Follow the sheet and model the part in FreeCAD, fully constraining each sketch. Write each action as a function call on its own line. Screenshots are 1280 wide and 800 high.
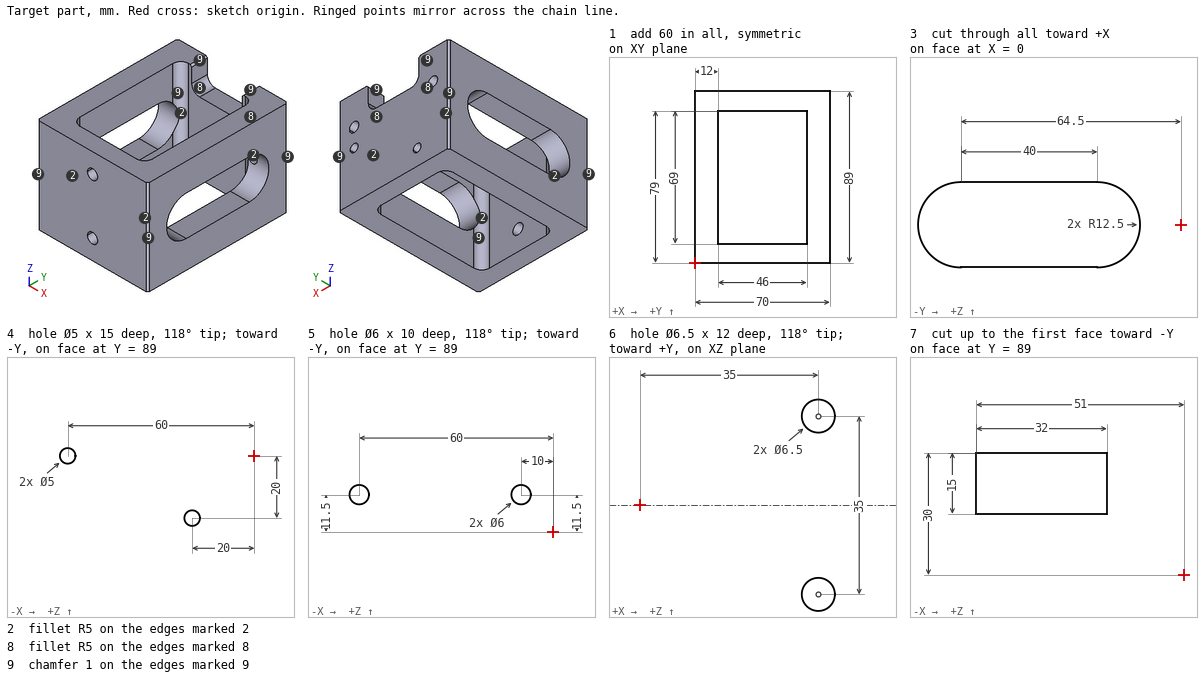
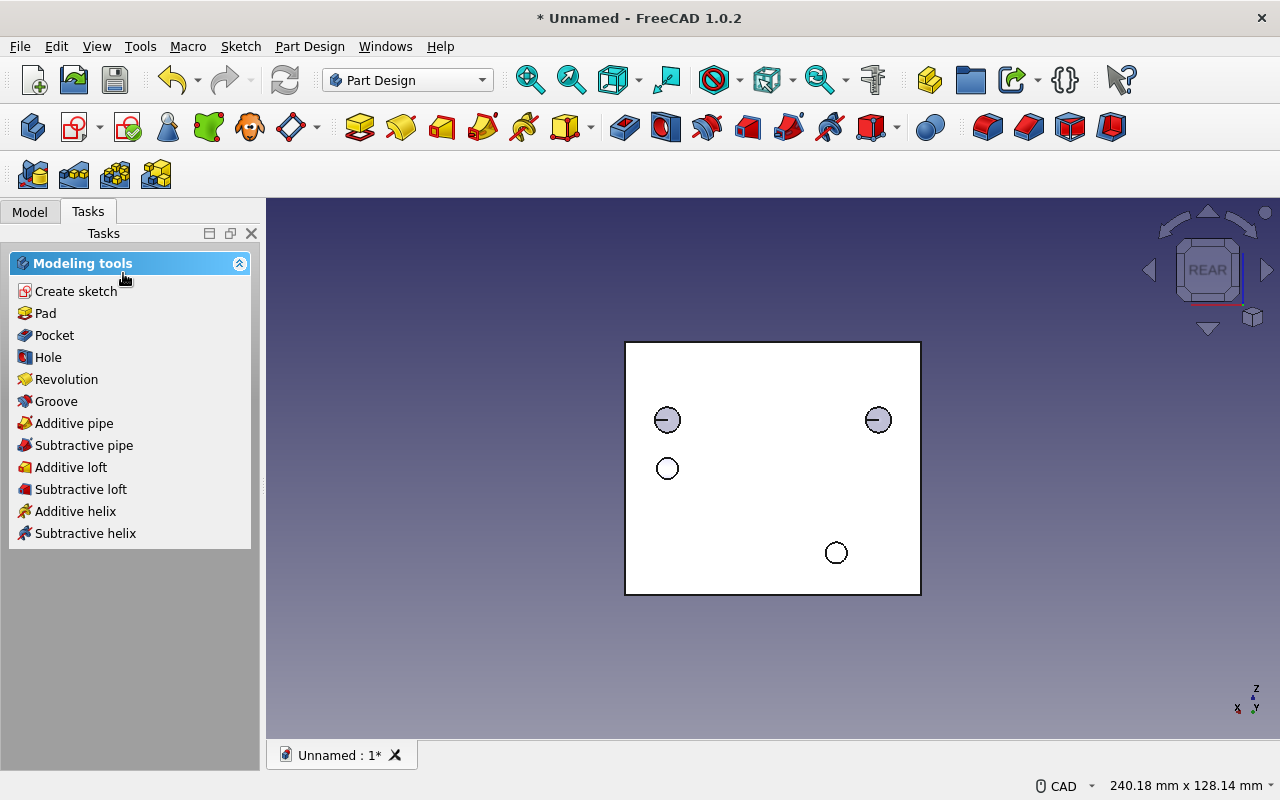
click(666, 128)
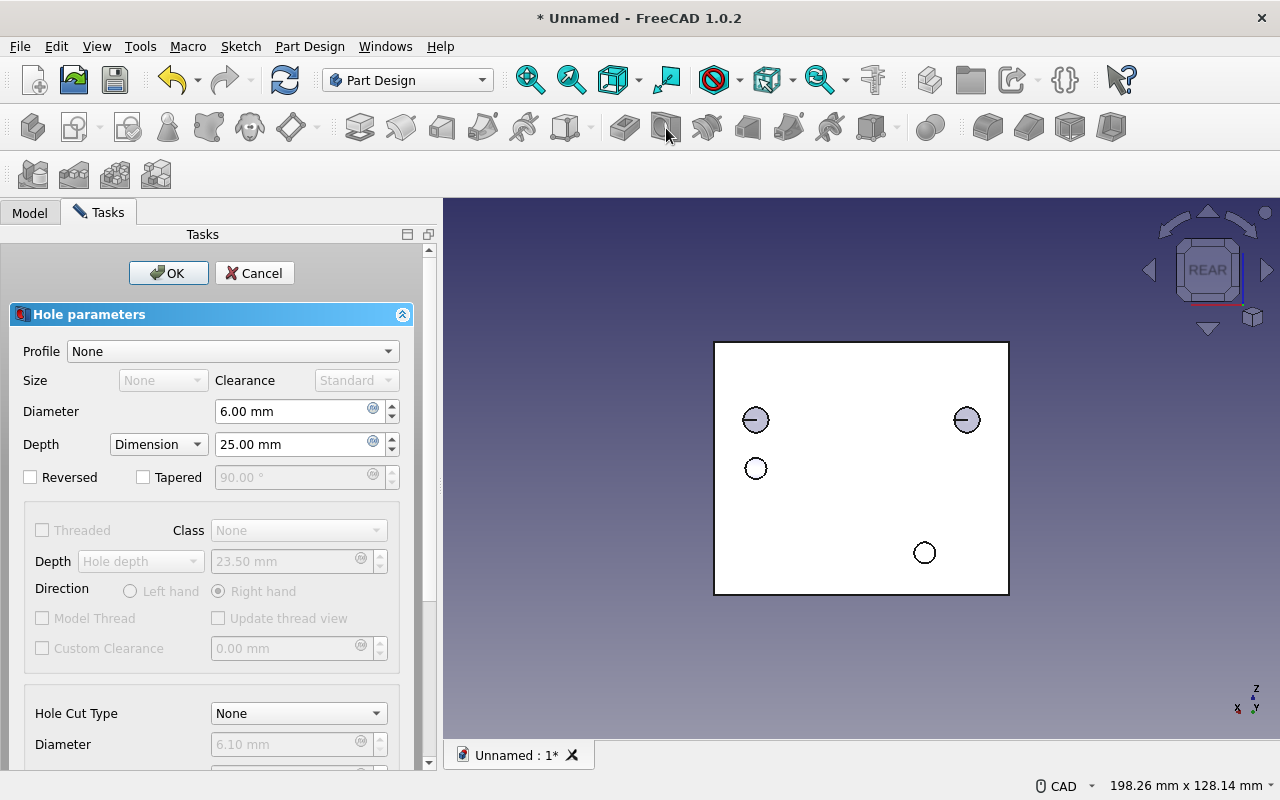
triple_click(300, 412)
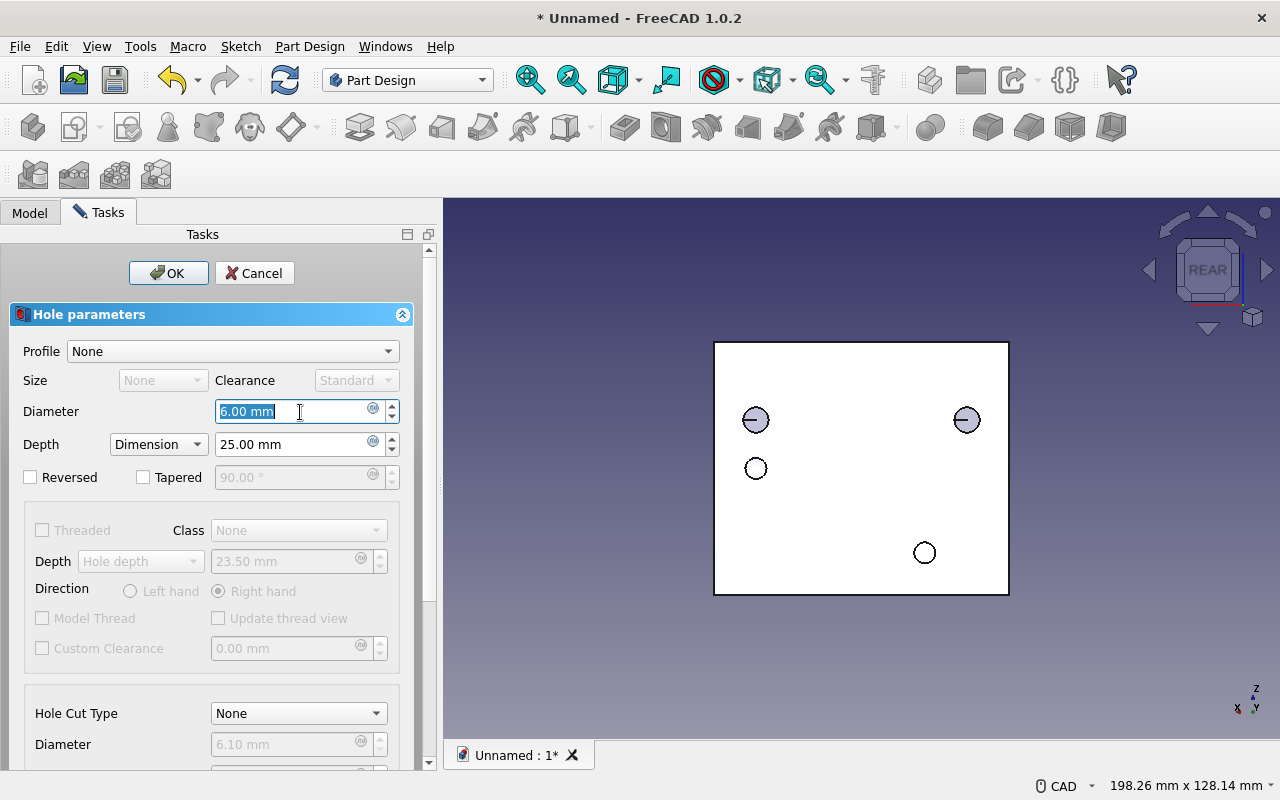
text(6.5)
key(Tab)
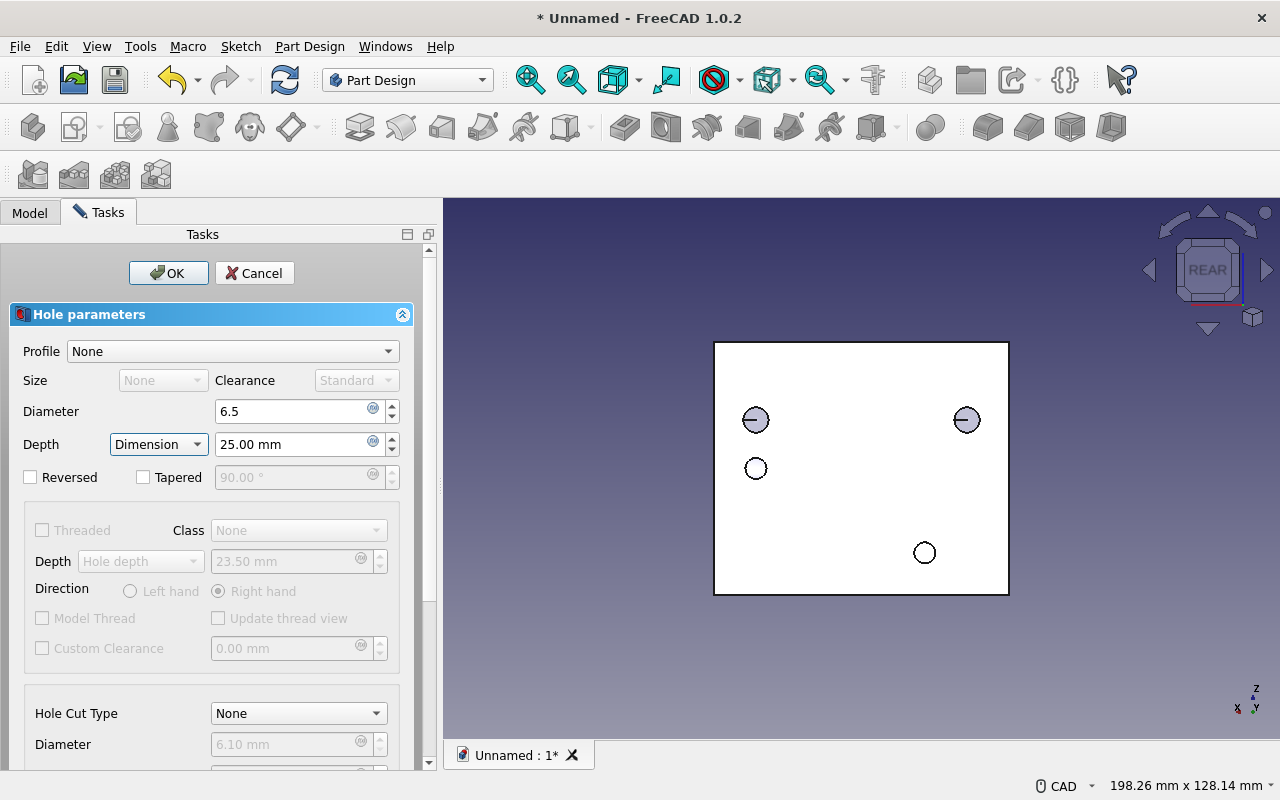
triple_click(300, 444)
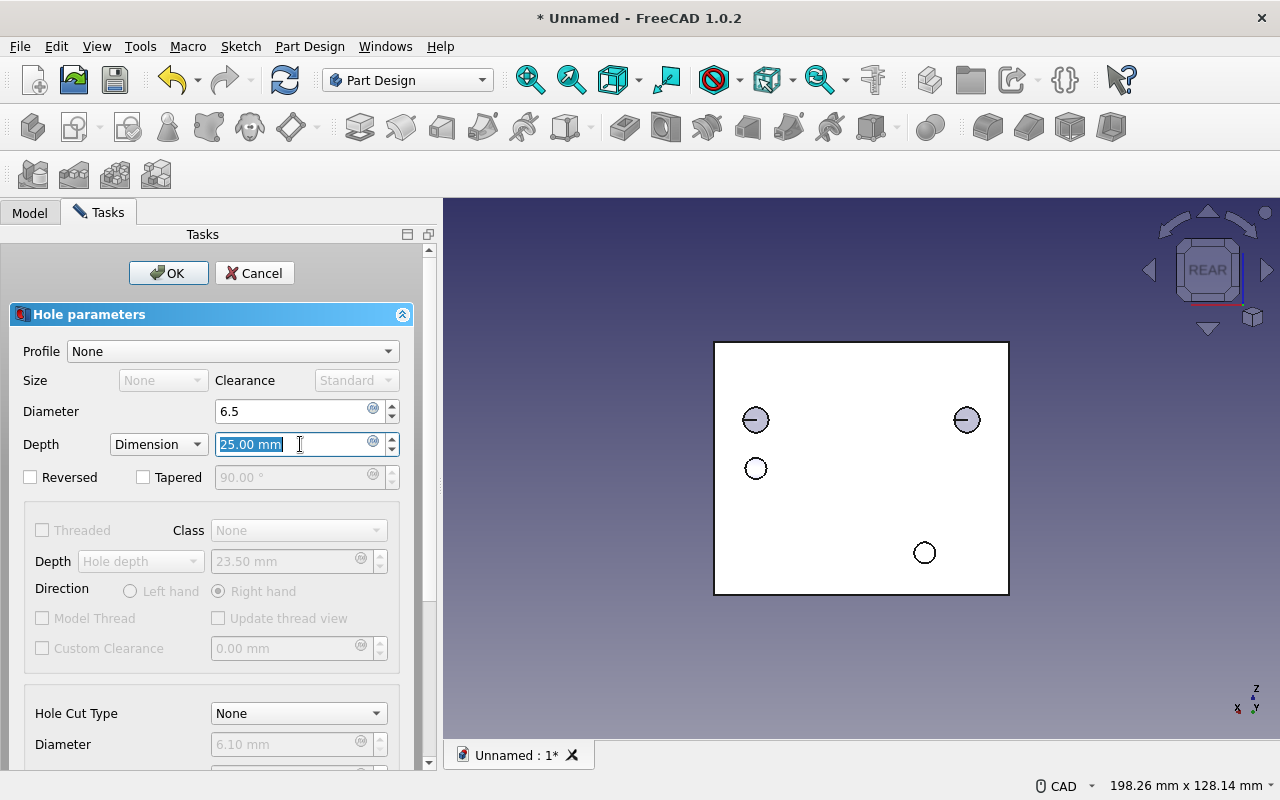
text(12)
key(Tab)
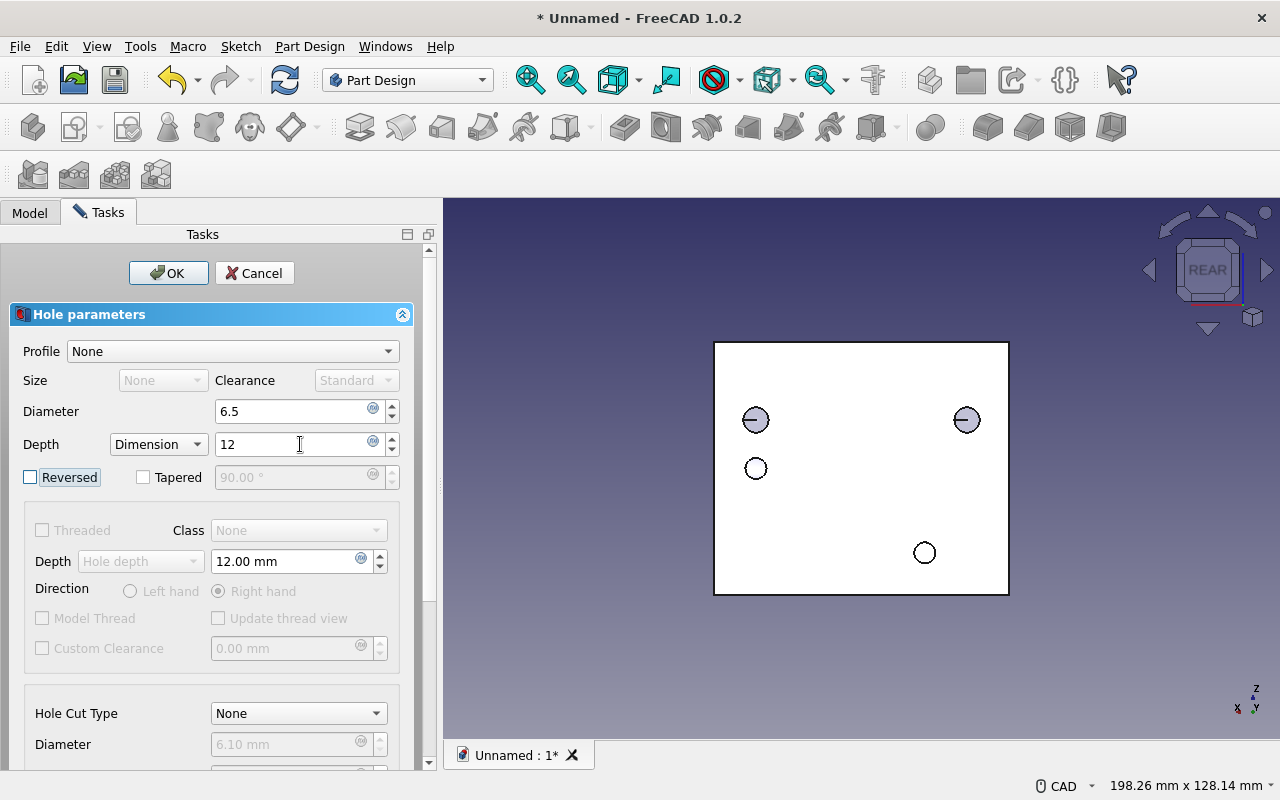
click(169, 273)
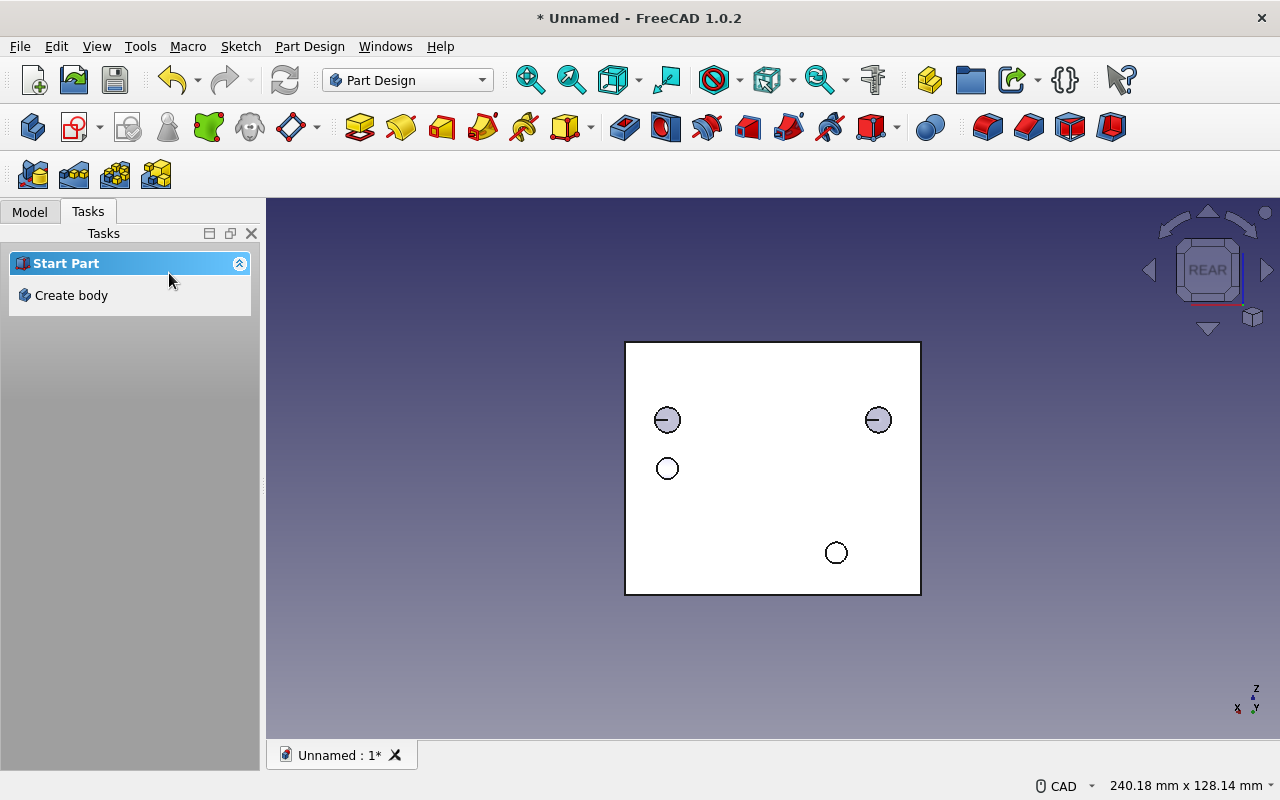
click(773, 468)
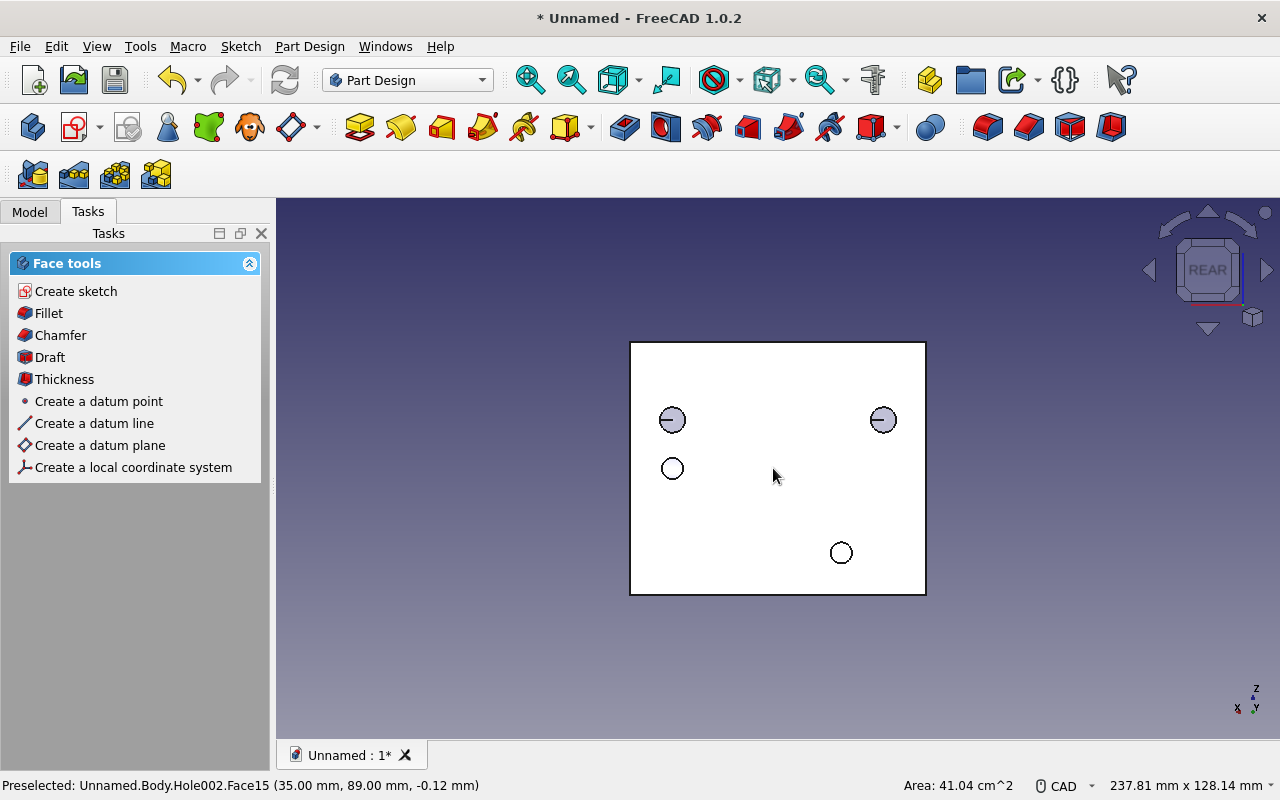
click(74, 128)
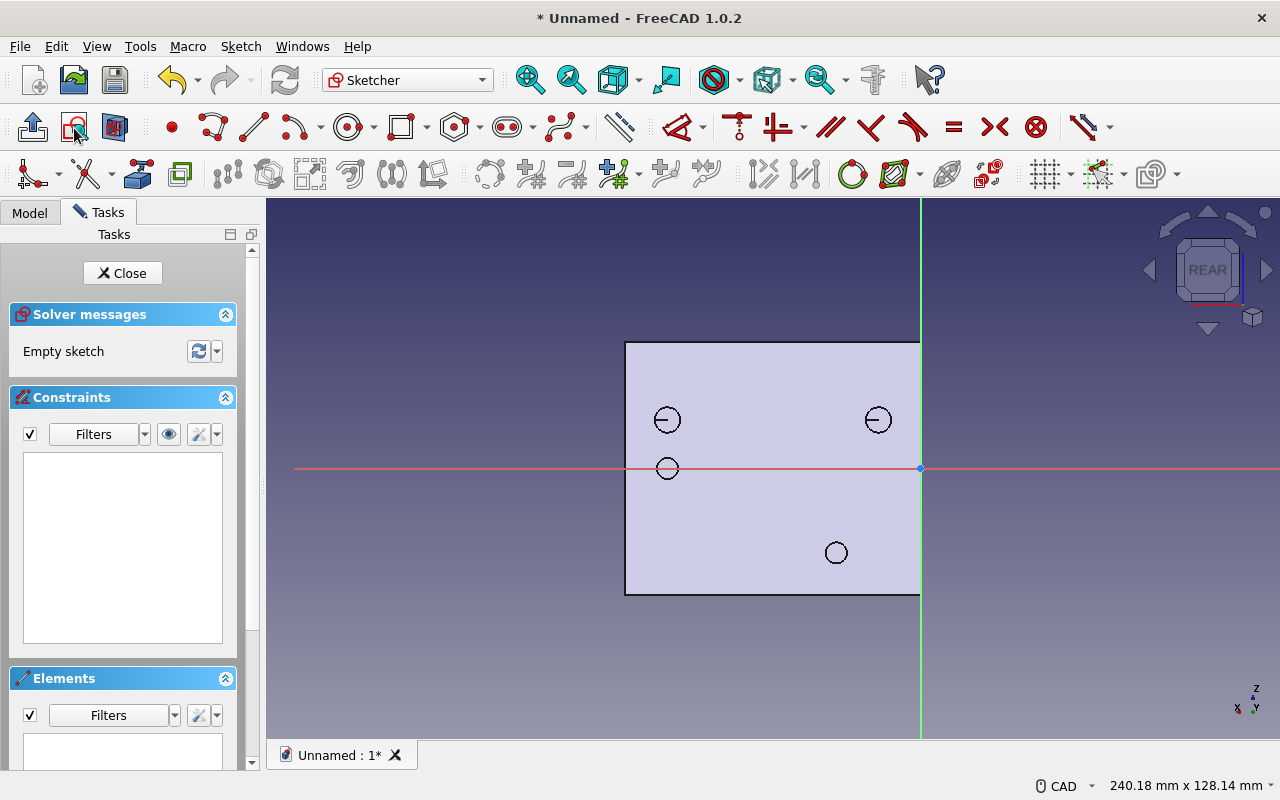
scroll(876, 368, up, 5)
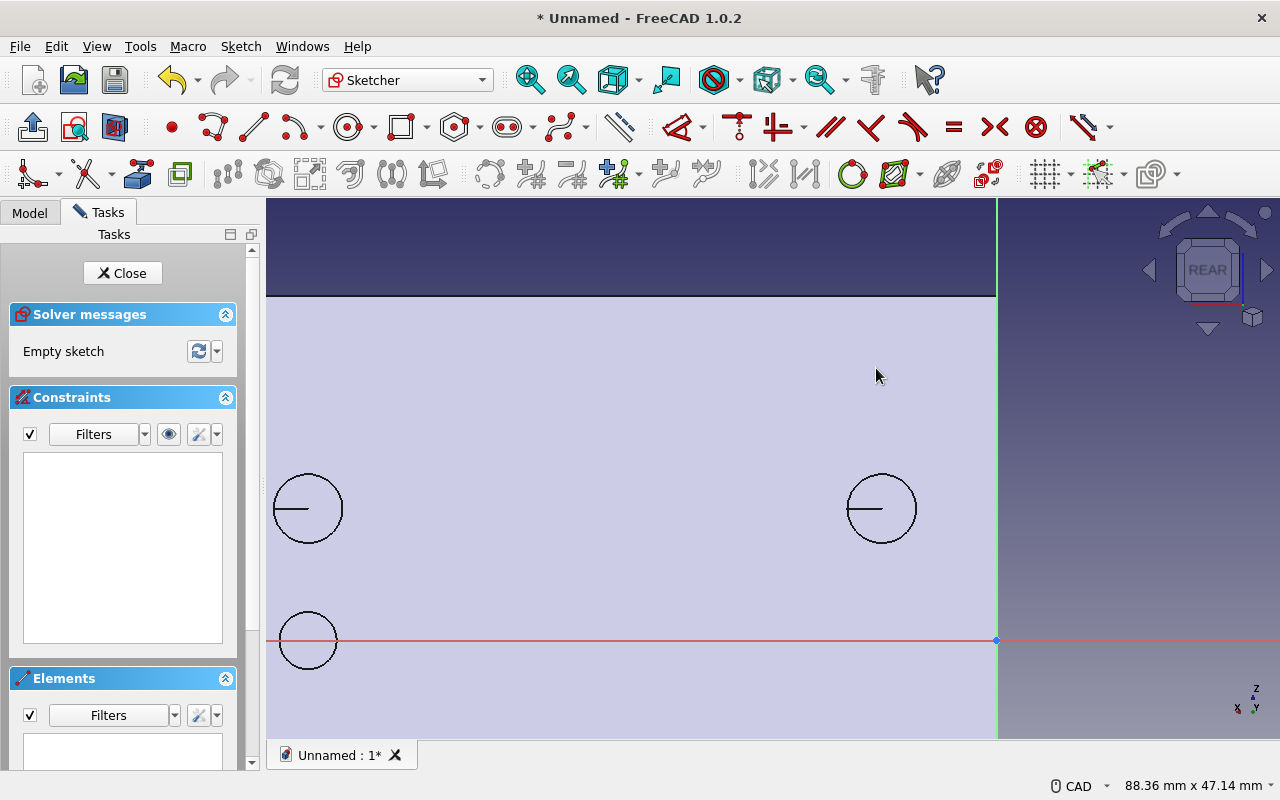
click(400, 128)